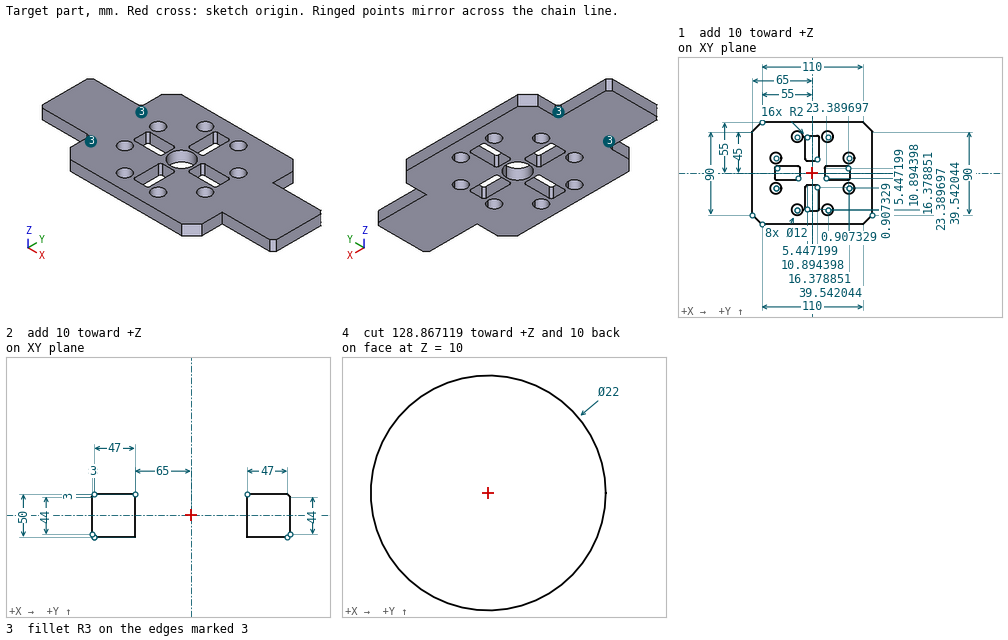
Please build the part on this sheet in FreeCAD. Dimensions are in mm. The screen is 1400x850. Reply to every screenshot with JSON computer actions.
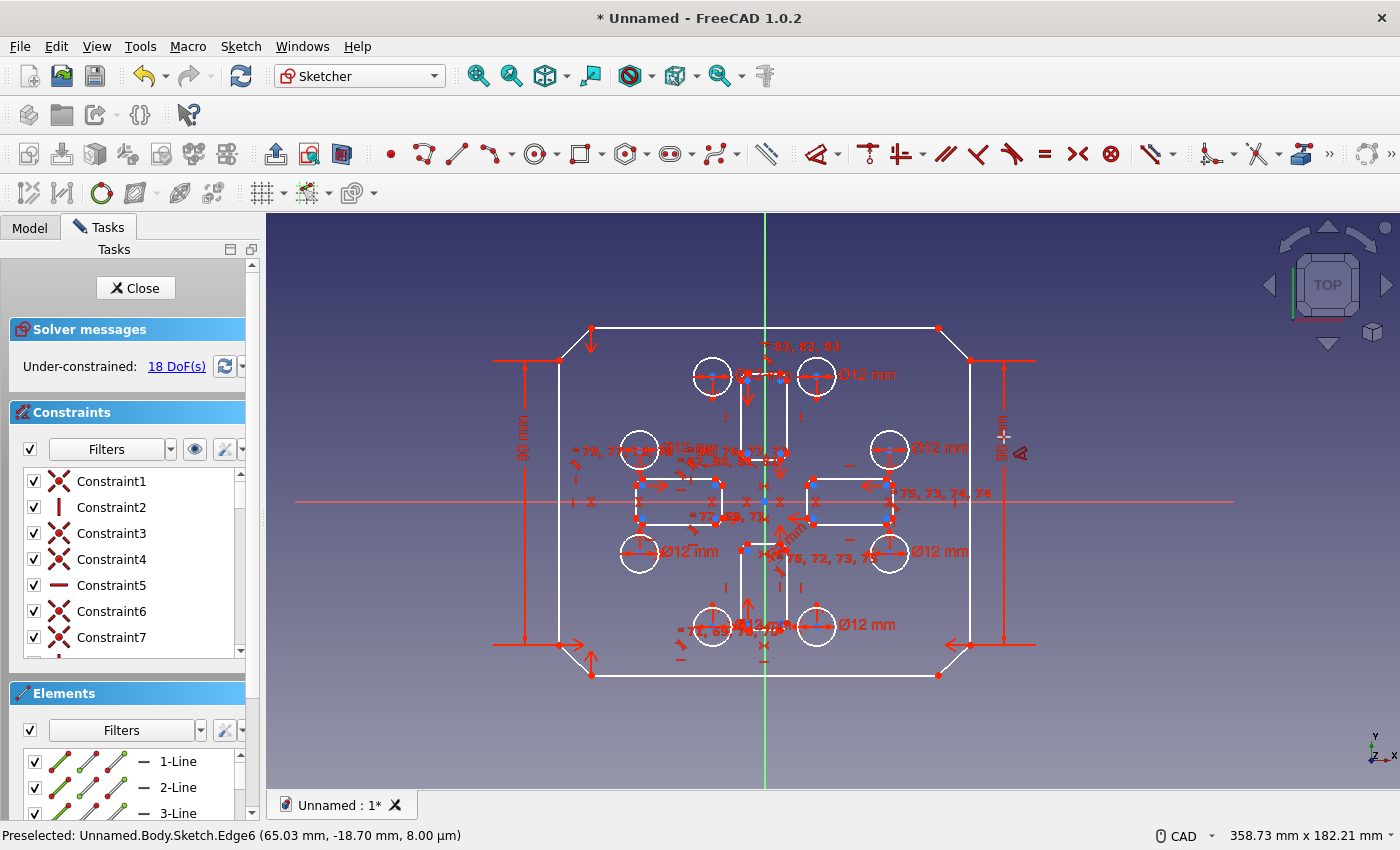
{"action": "left_click", "coordinate": [695, 675]}
{"action": "left_click", "coordinate": [685, 709]}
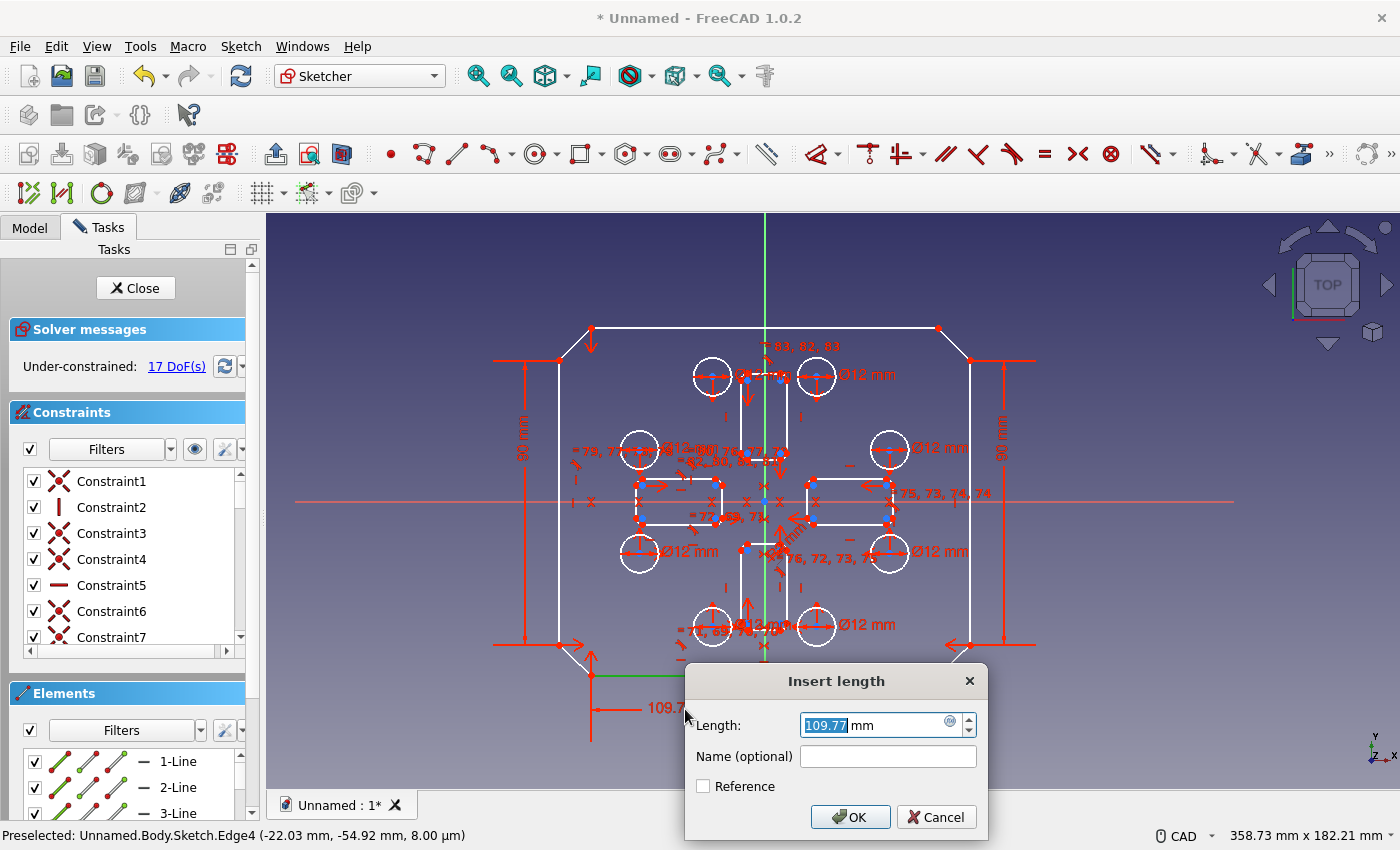
{"action": "type", "text": "110"}
{"action": "key", "text": "Return"}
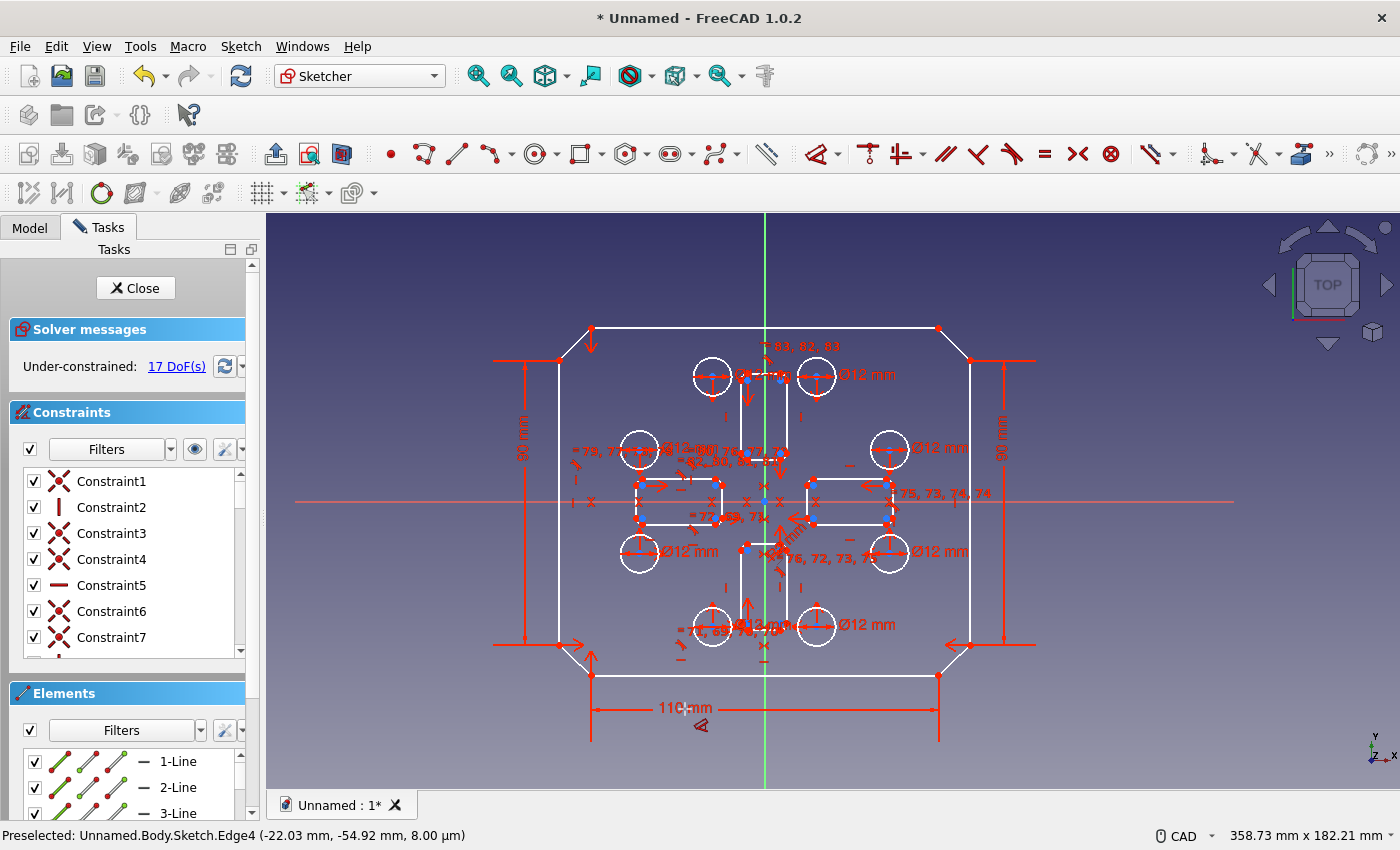
{"action": "left_click", "coordinate": [834, 328]}
{"action": "left_click", "coordinate": [685, 294]}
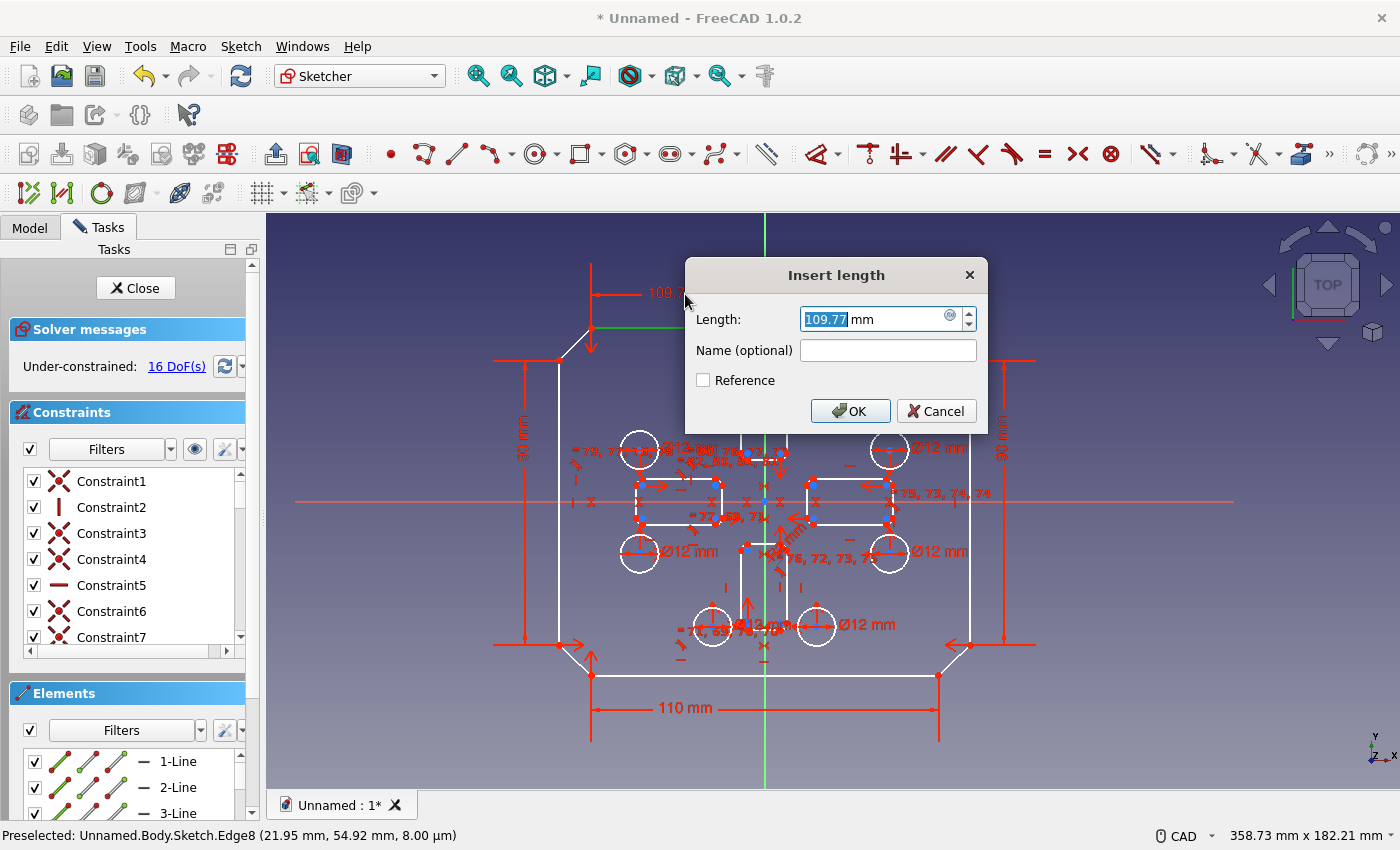
{"action": "type", "text": "110"}
{"action": "key", "text": "Return"}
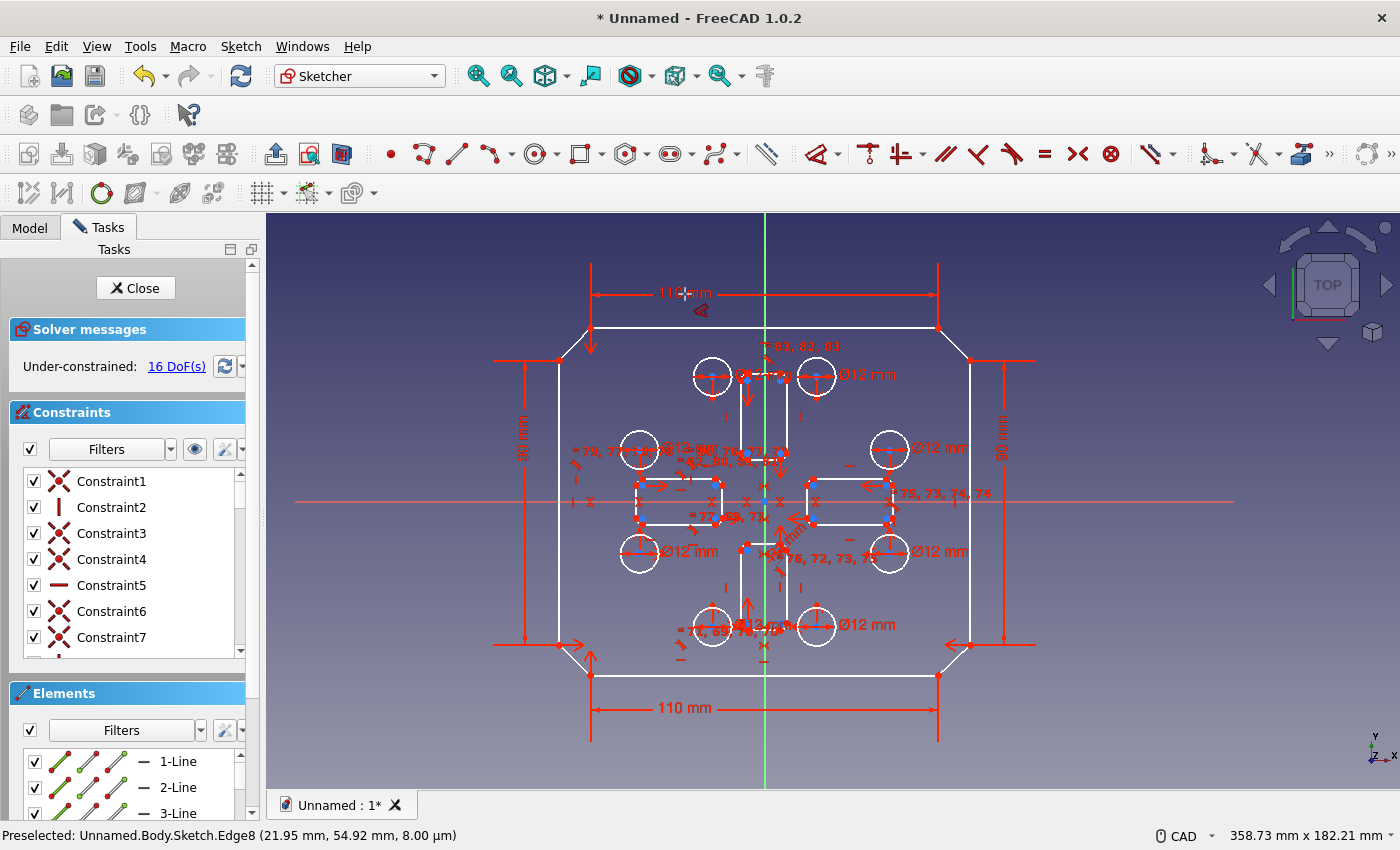
{"action": "left_click", "coordinate": [591, 328]}
{"action": "left_click", "coordinate": [678, 270]}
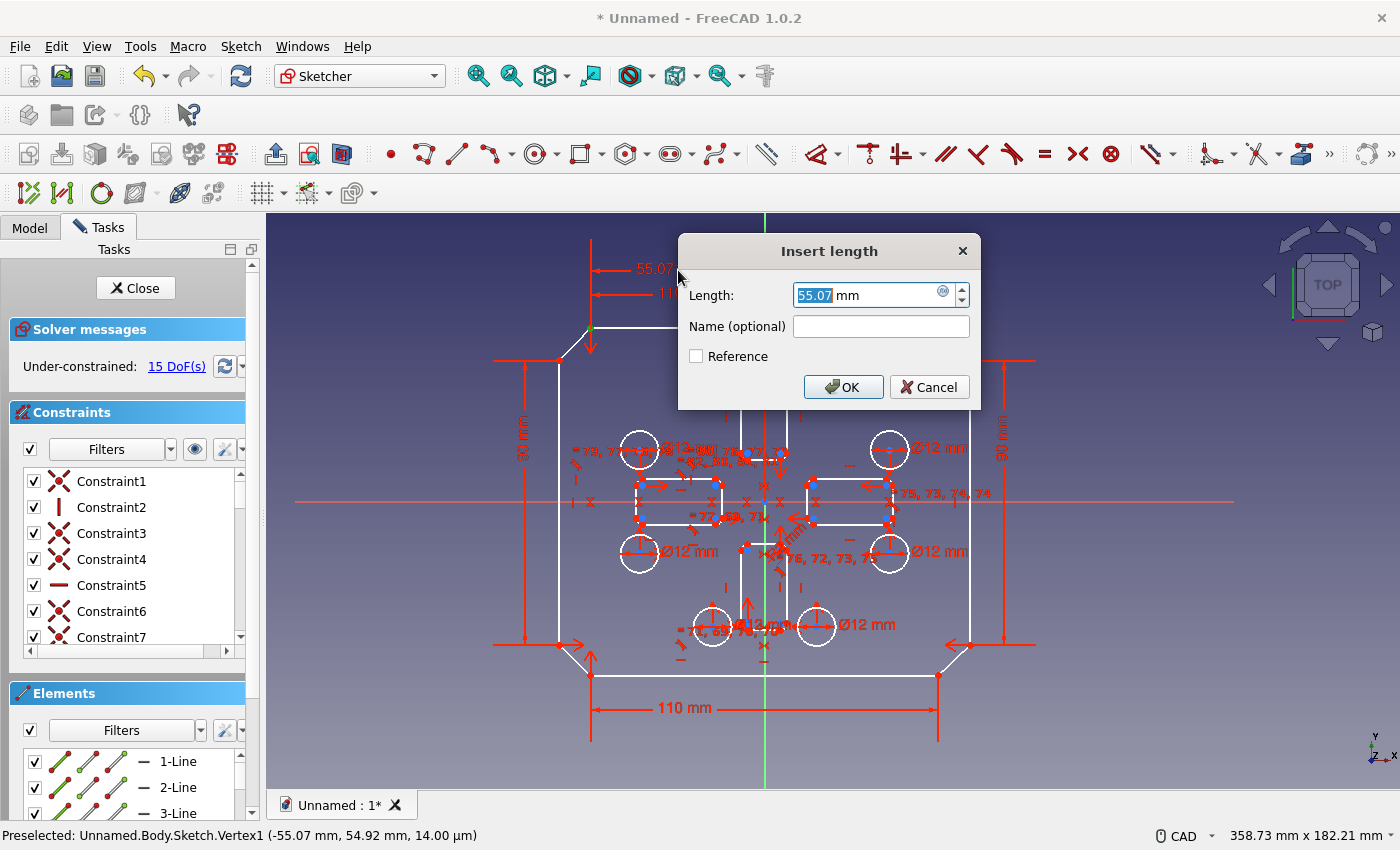
{"action": "type", "text": "55"}
{"action": "key", "text": "Return"}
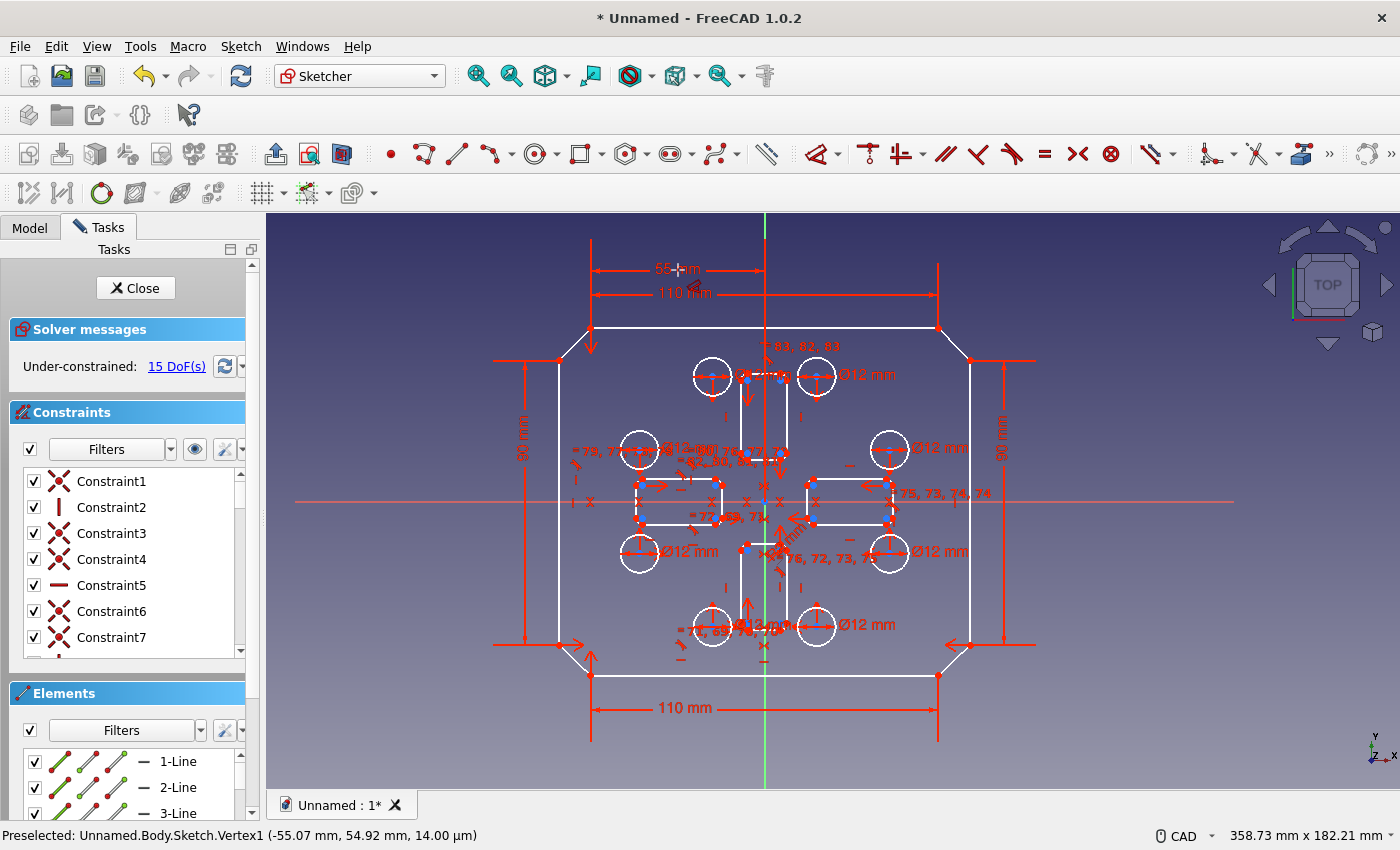
{"action": "left_click", "coordinate": [591, 328]}
{"action": "left_click", "coordinate": [533, 415]}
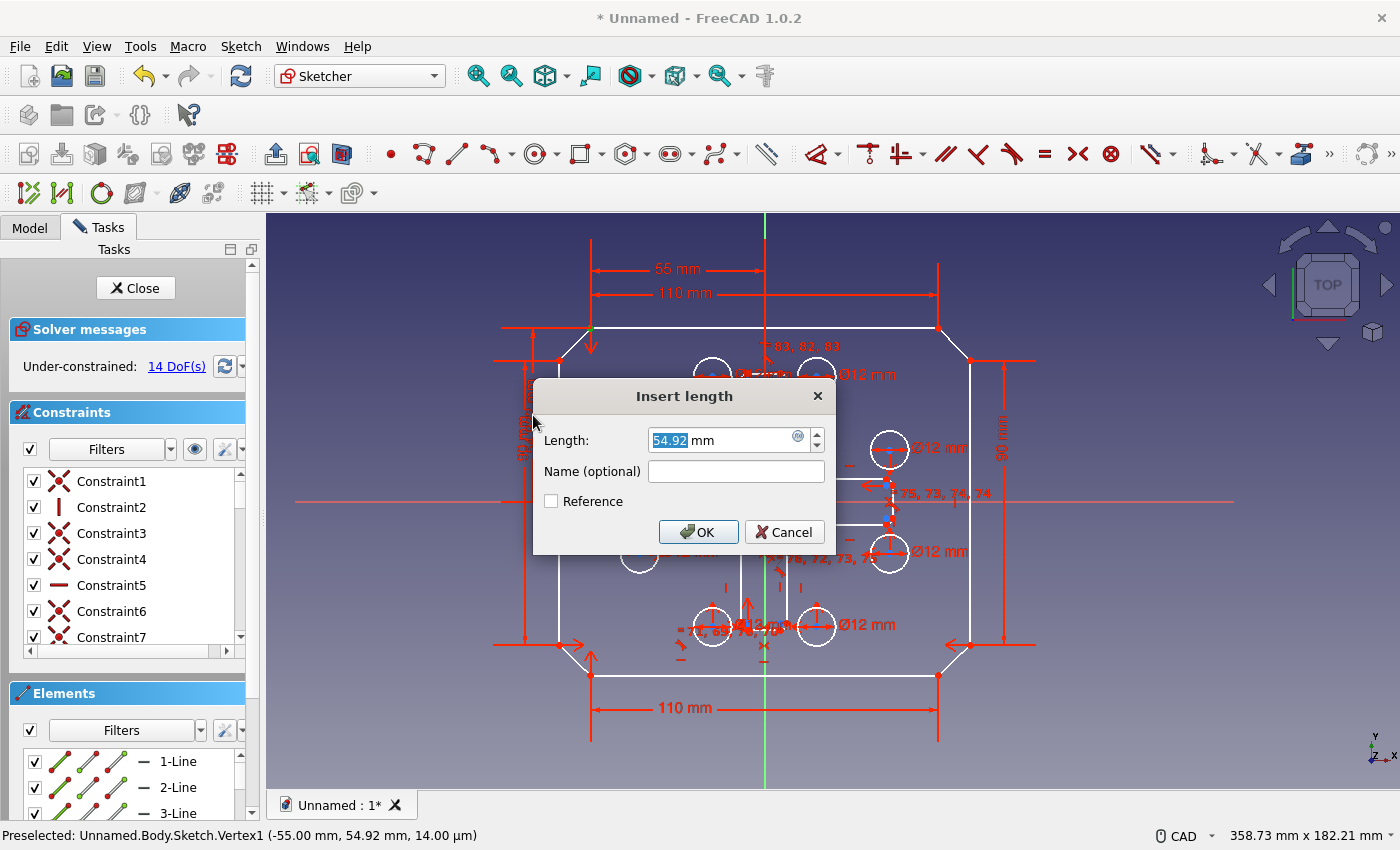
{"action": "type", "text": "55"}
{"action": "key", "text": "Return"}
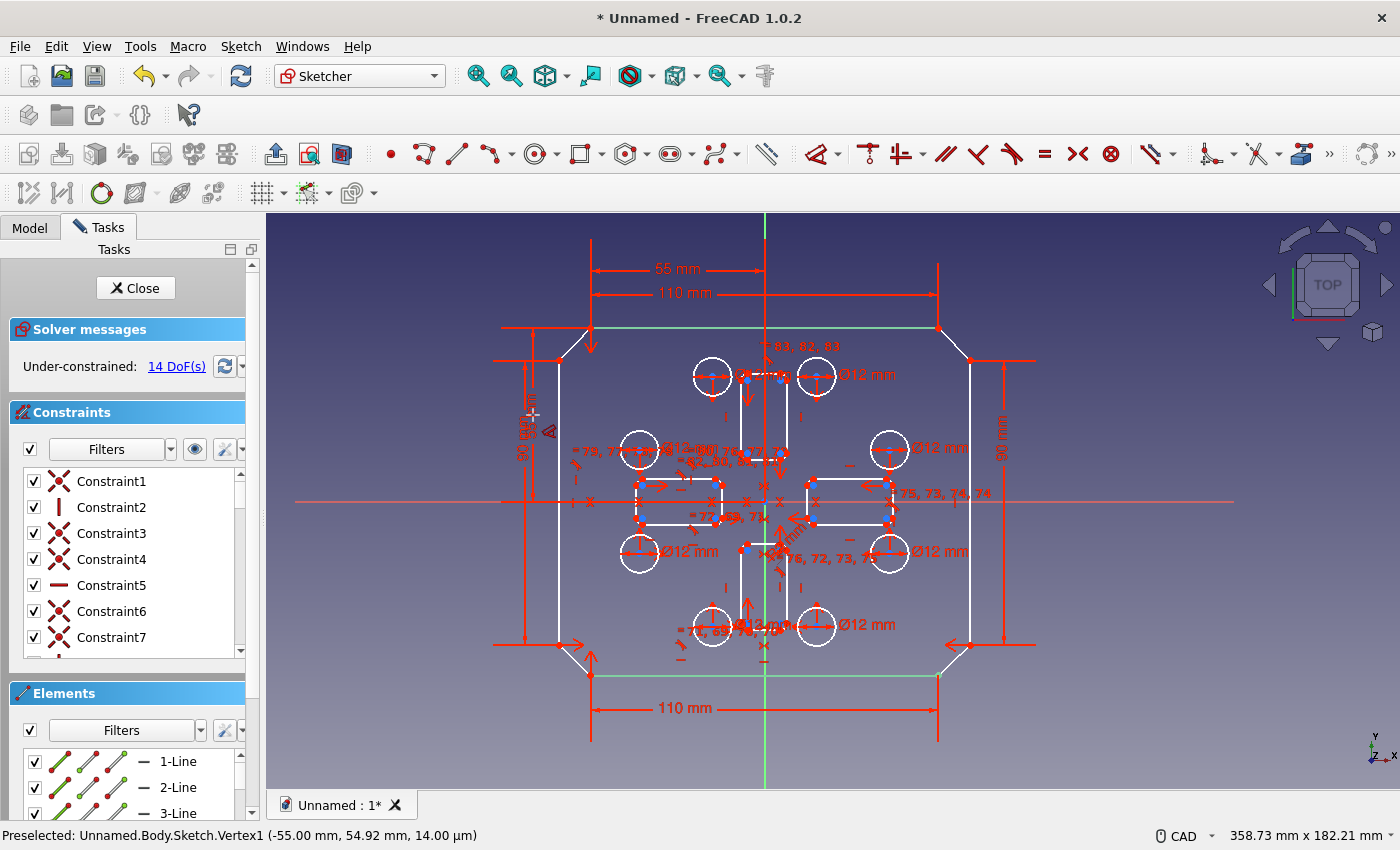
{"action": "left_click", "coordinate": [559, 361]}
{"action": "left_click", "coordinate": [590, 536]}